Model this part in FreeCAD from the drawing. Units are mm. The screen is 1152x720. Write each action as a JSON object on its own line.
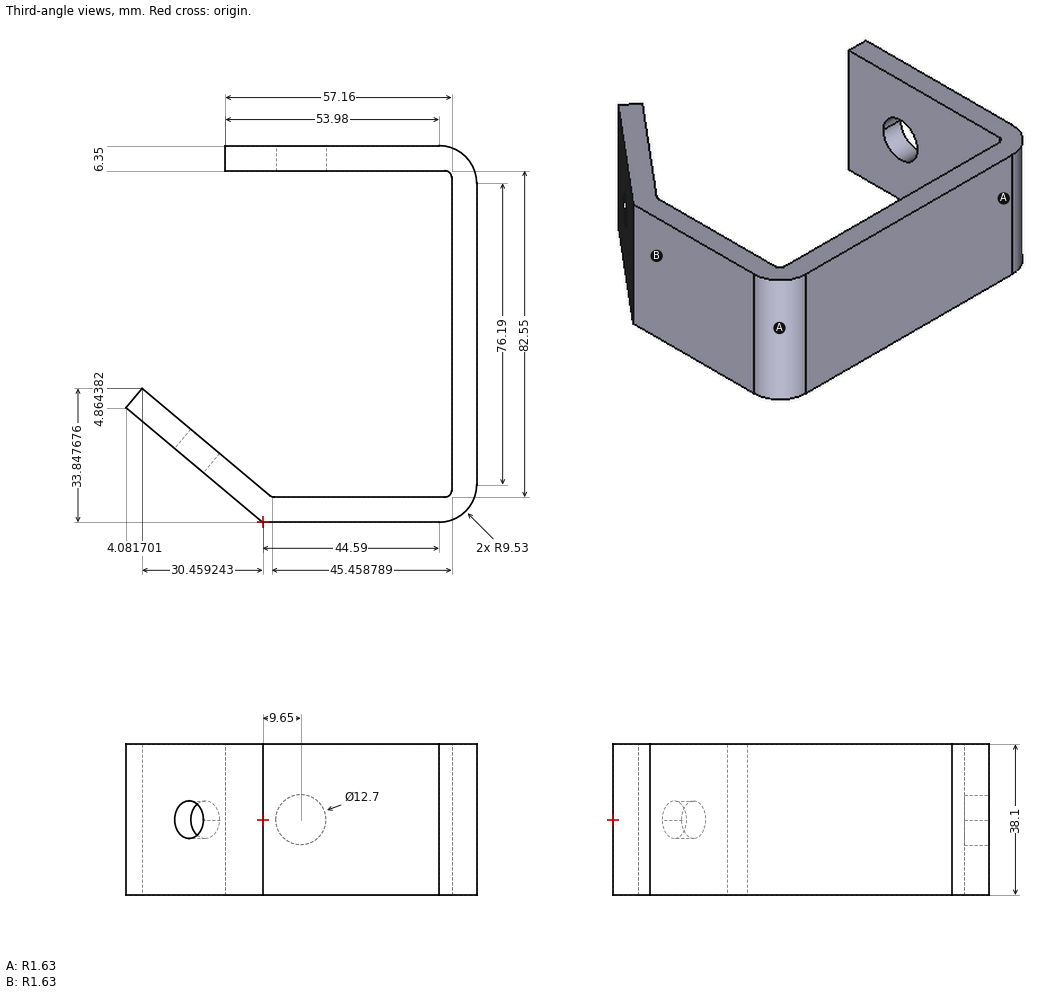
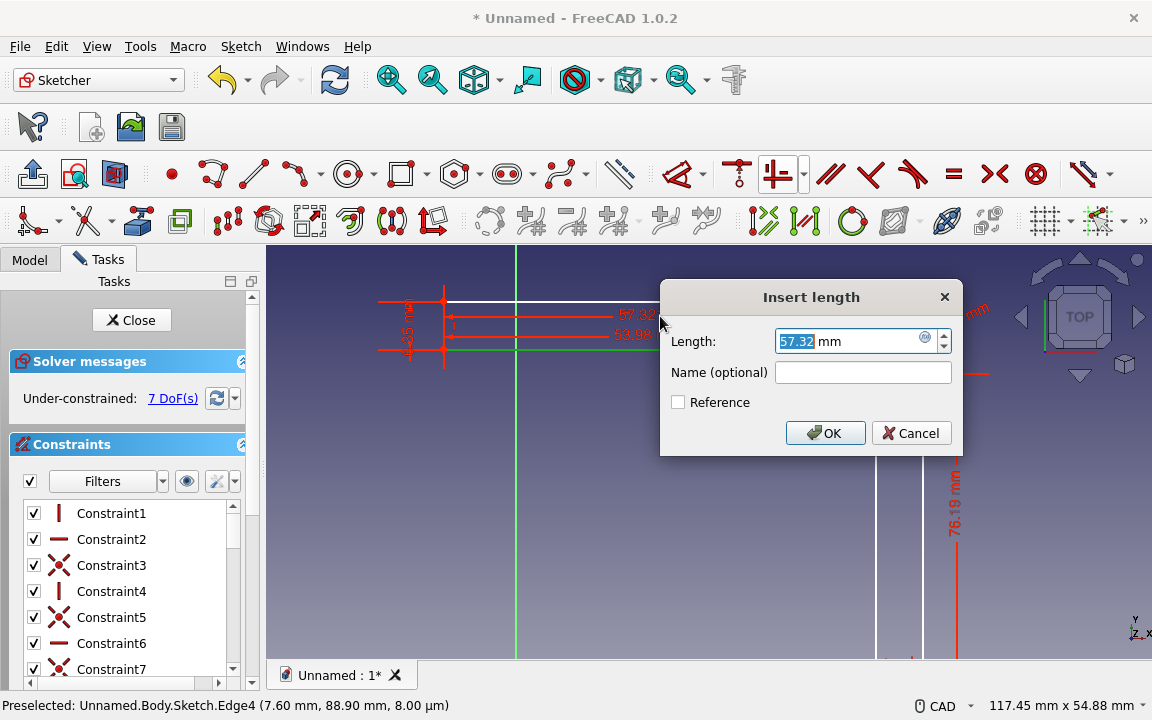
{"action": "type", "text": "57.16"}
{"action": "key", "text": "Return"}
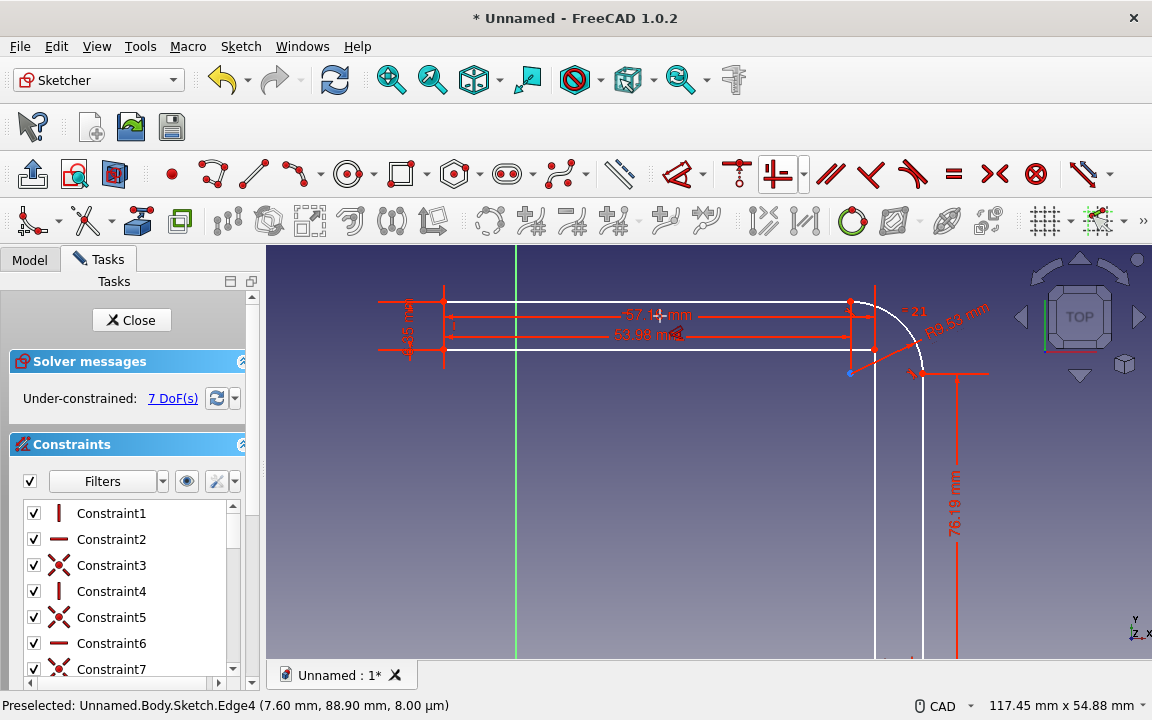
{"action": "left_click", "coordinate": [875, 538]}
{"action": "left_click", "coordinate": [909, 426]}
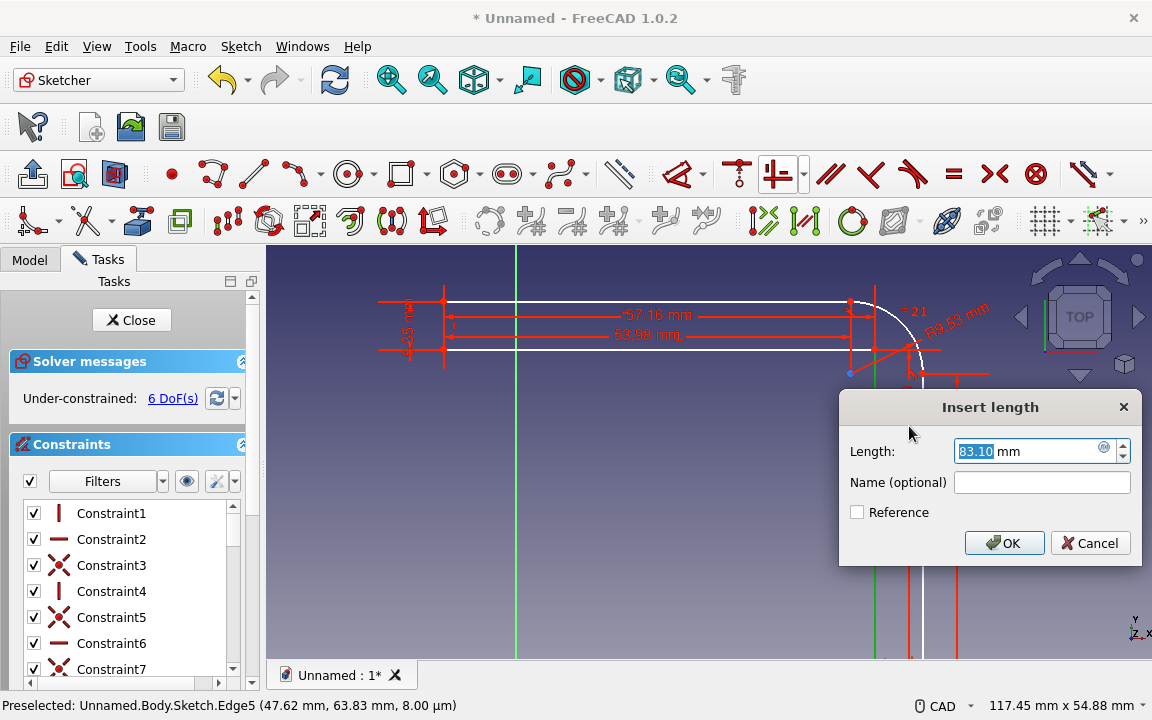
{"action": "type", "text": "82.55"}
{"action": "key", "text": "Return"}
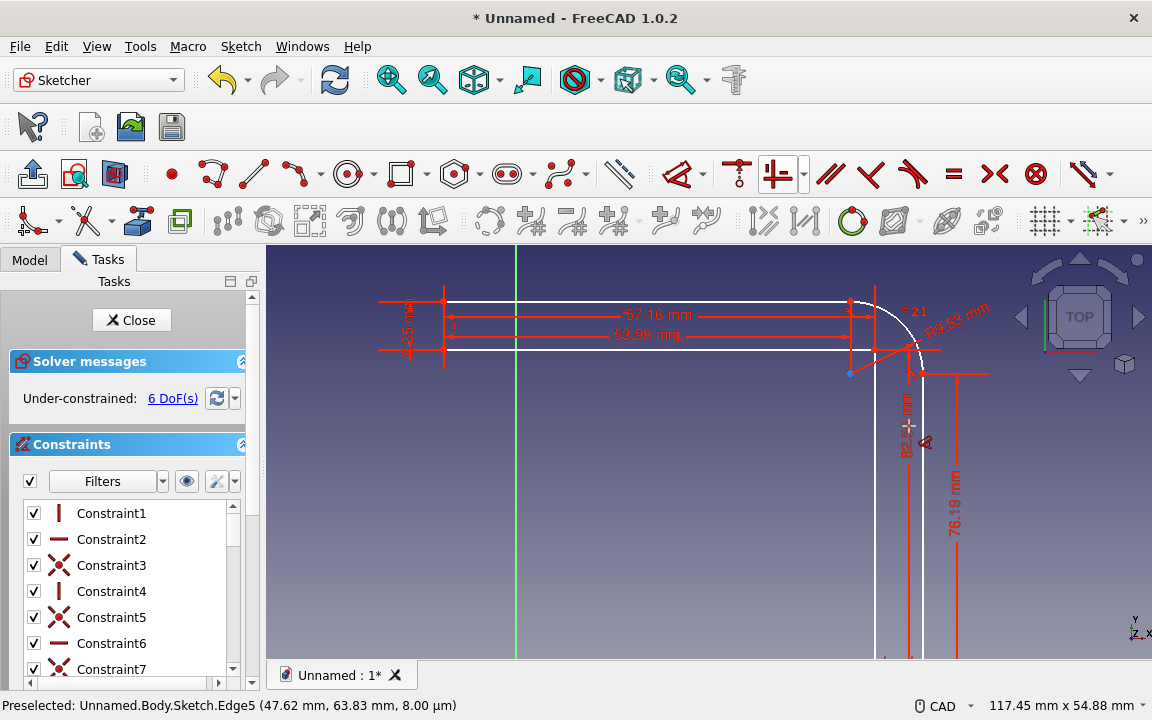
{"action": "scroll", "coordinate": [670, 330], "scroll_direction": "down", "scroll_amount": 5}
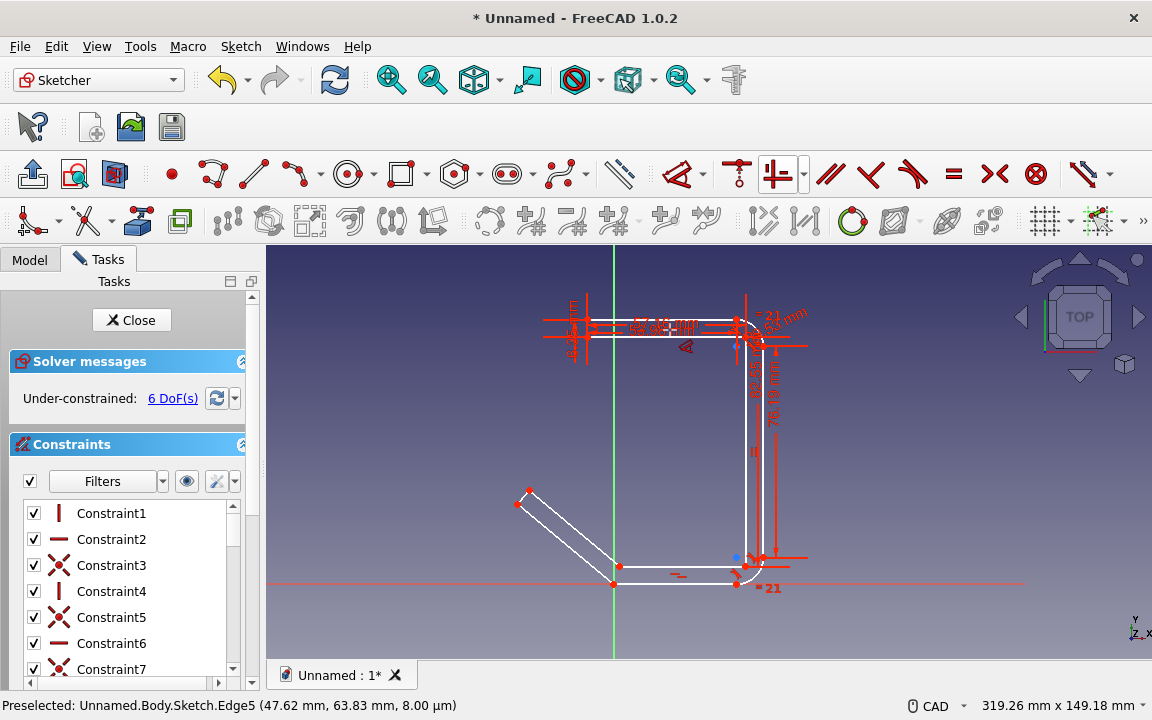
{"action": "left_click", "coordinate": [651, 584]}
{"action": "left_click", "coordinate": [675, 618]}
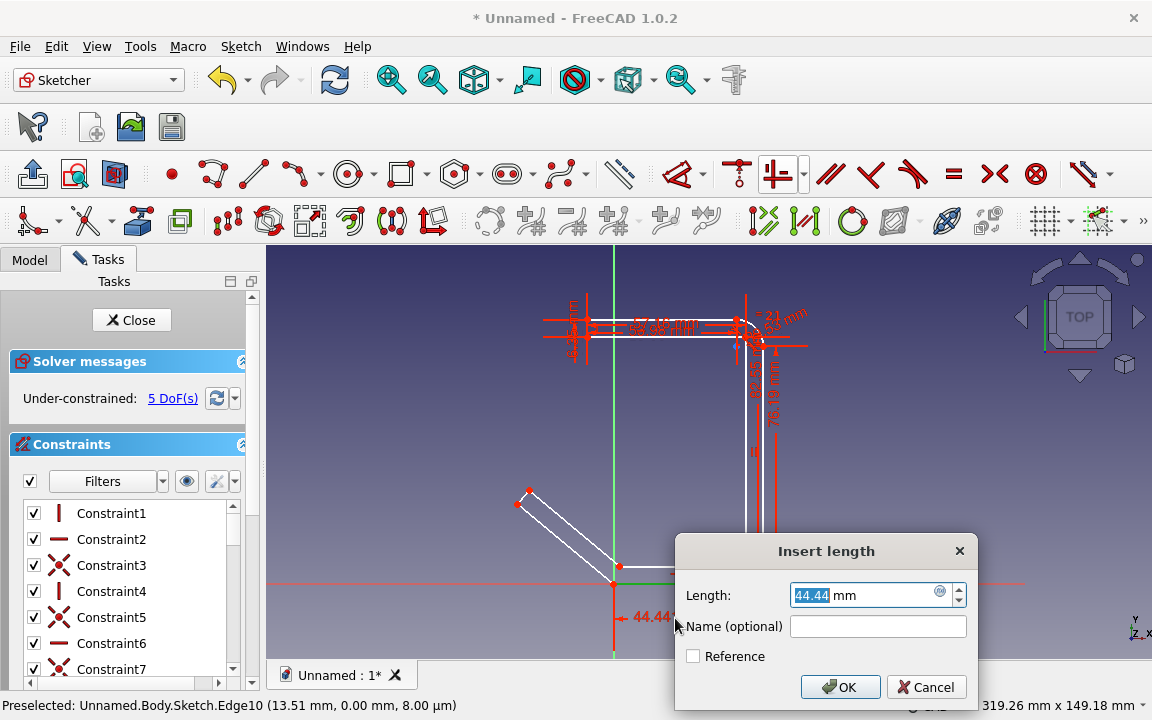
{"action": "type", "text": "44.59"}
{"action": "key", "text": "Return"}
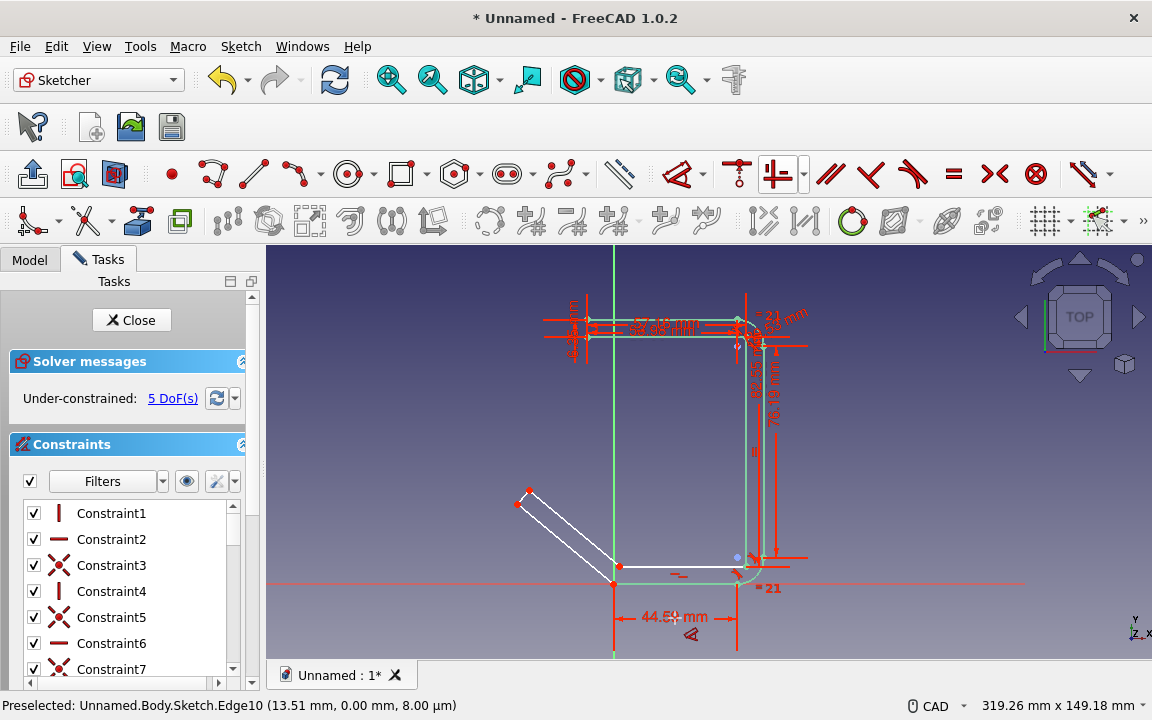
{"action": "left_click", "coordinate": [708, 567]}
{"action": "left_click", "coordinate": [683, 533]}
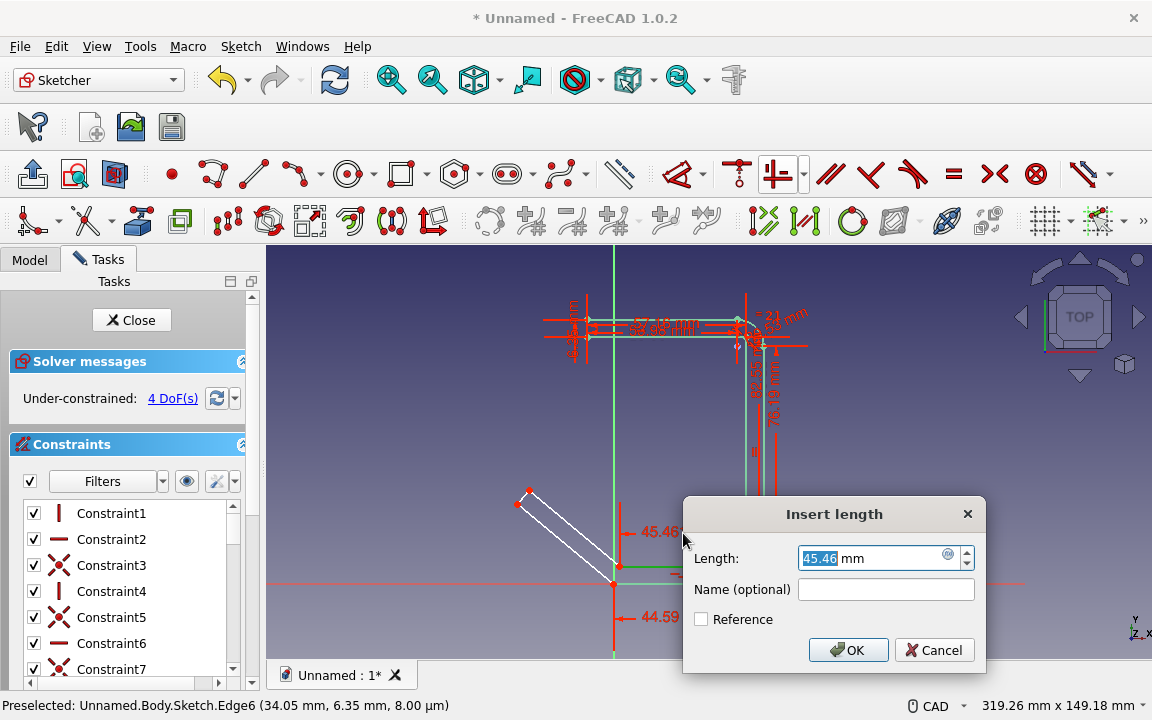
{"action": "type", "text": "45.458789"}
{"action": "key", "text": "Return"}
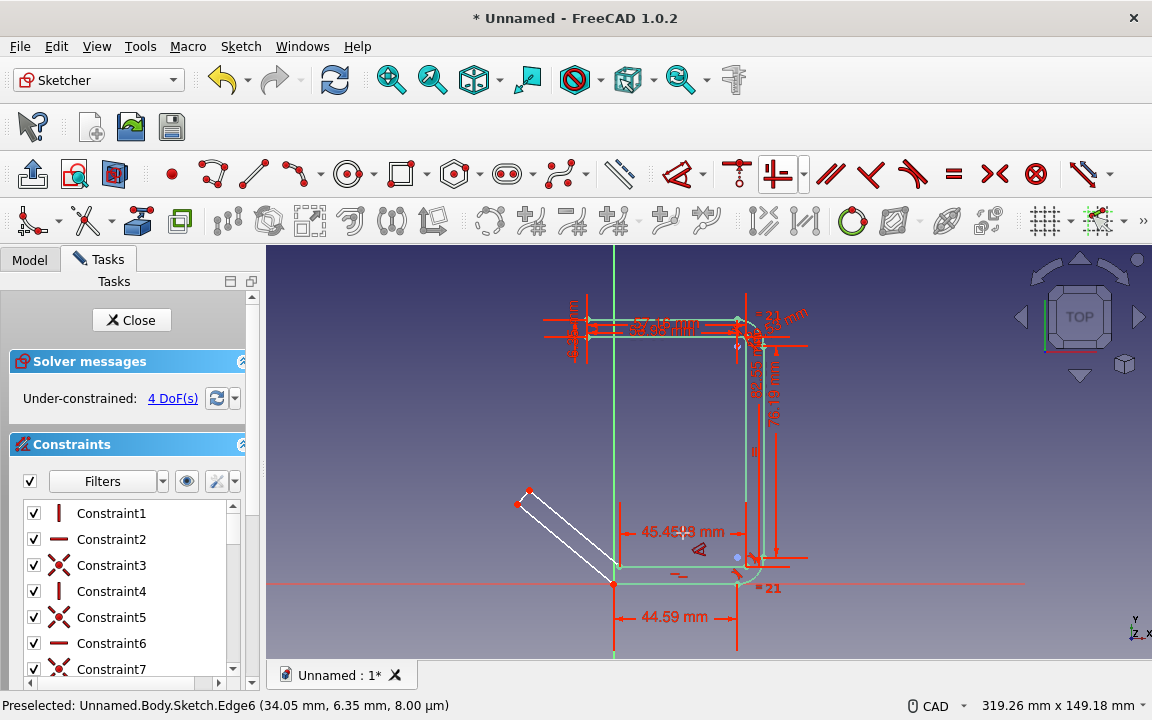
{"action": "scroll", "coordinate": [523, 497], "scroll_direction": "up", "scroll_amount": 7}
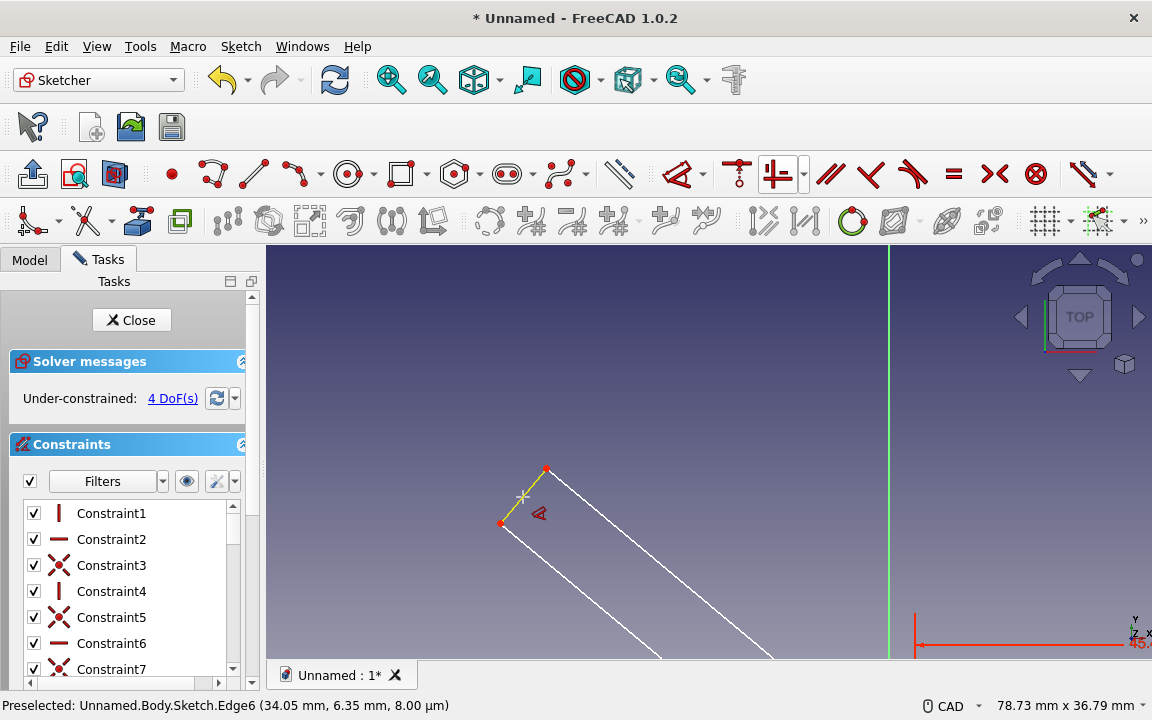
{"action": "left_click", "coordinate": [524, 496]}
{"action": "left_click", "coordinate": [513, 558]}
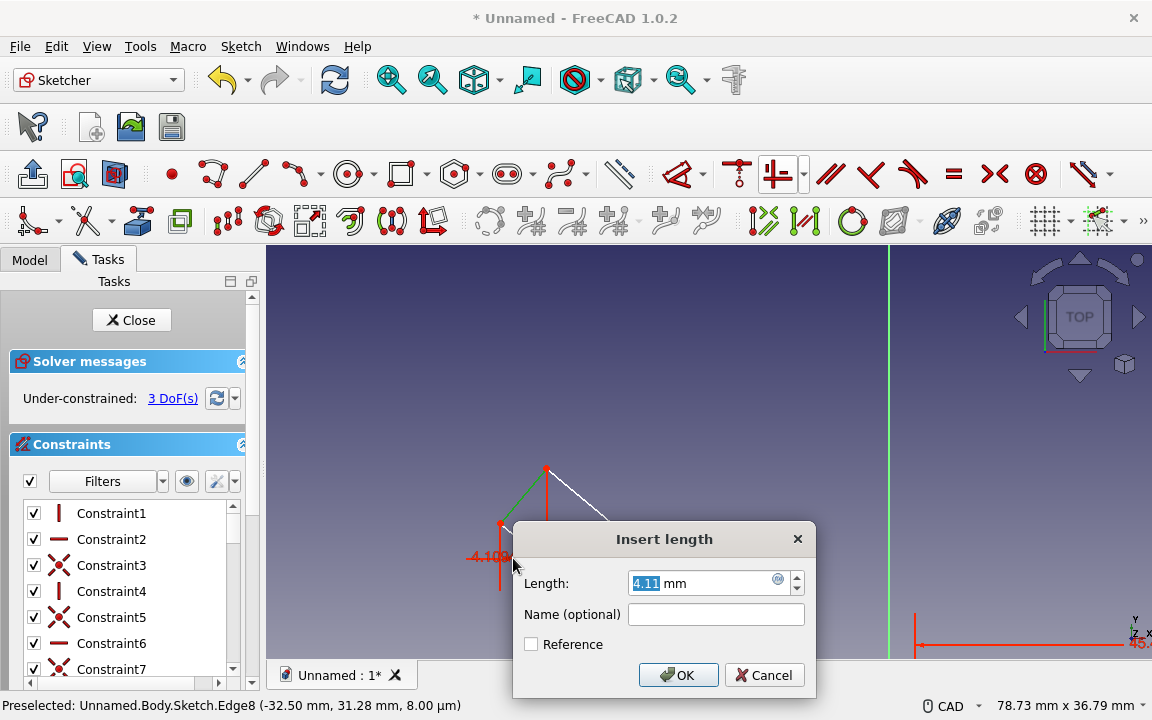
{"action": "type", "text": "4.081701"}
{"action": "key", "text": "Return"}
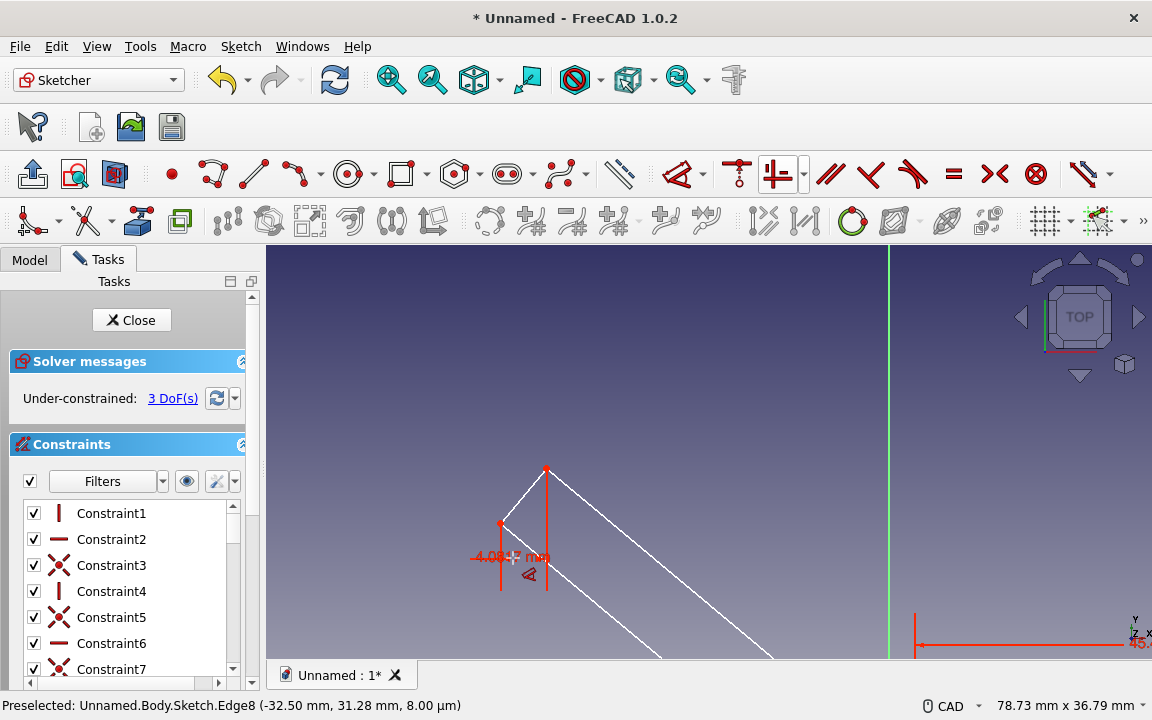
{"action": "left_click", "coordinate": [533, 485]}
{"action": "left_click", "coordinate": [467, 496]}